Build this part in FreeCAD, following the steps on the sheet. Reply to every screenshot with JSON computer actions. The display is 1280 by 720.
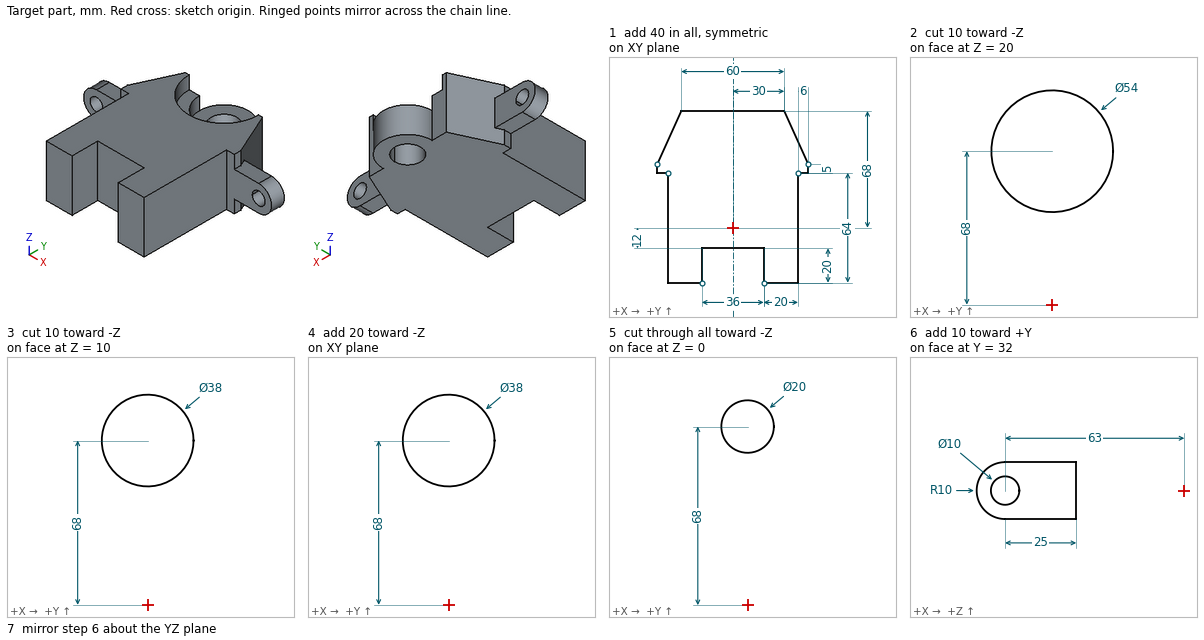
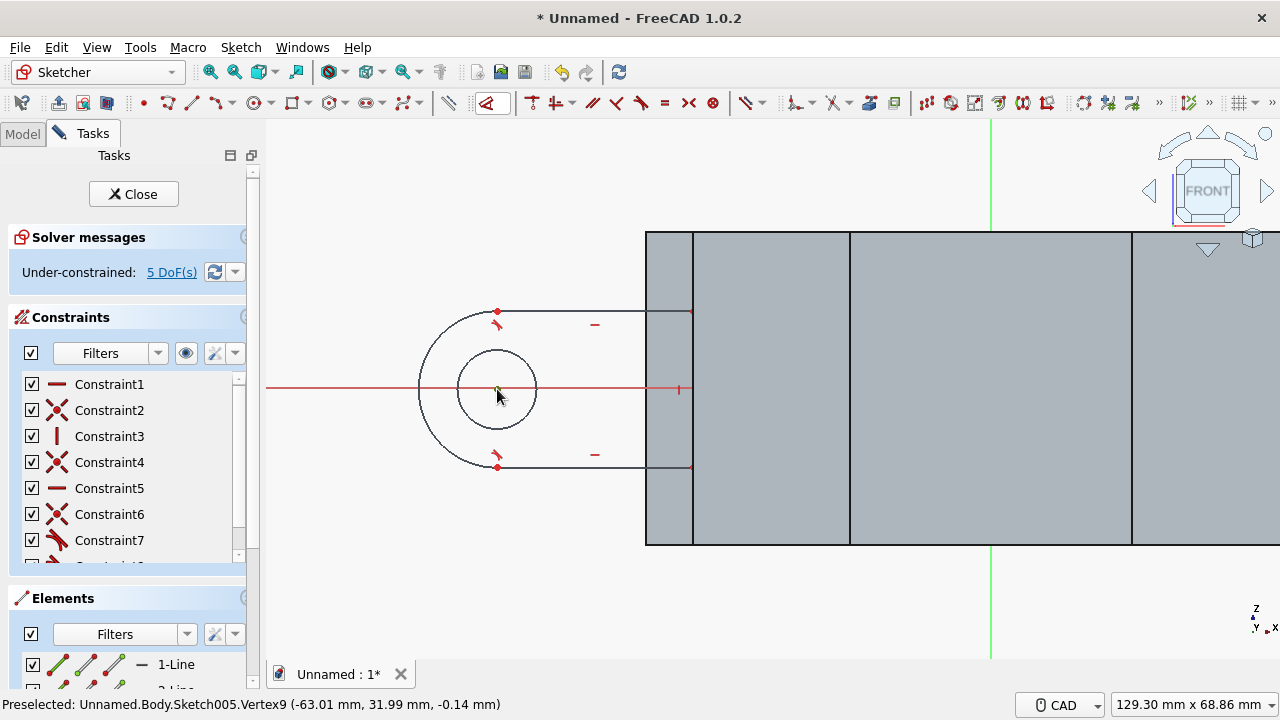
{"action": "left_click", "coordinate": [353, 388]}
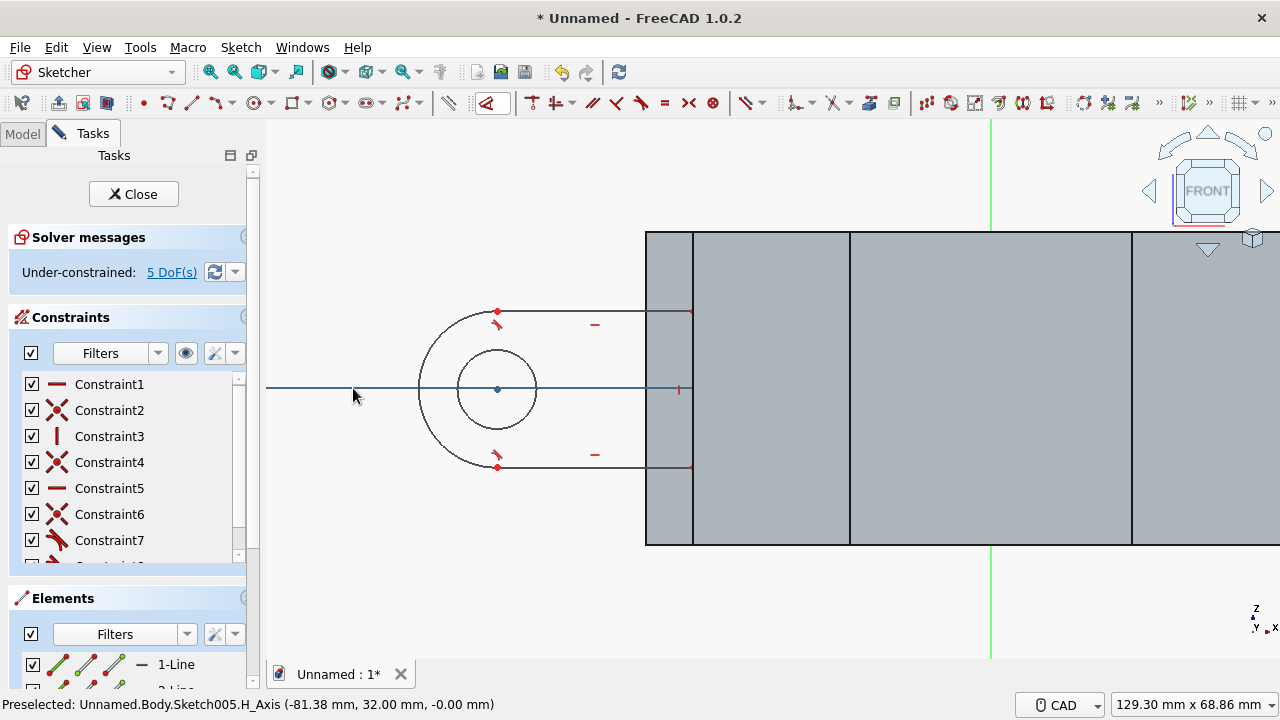
{"action": "left_click", "coordinate": [532, 104]}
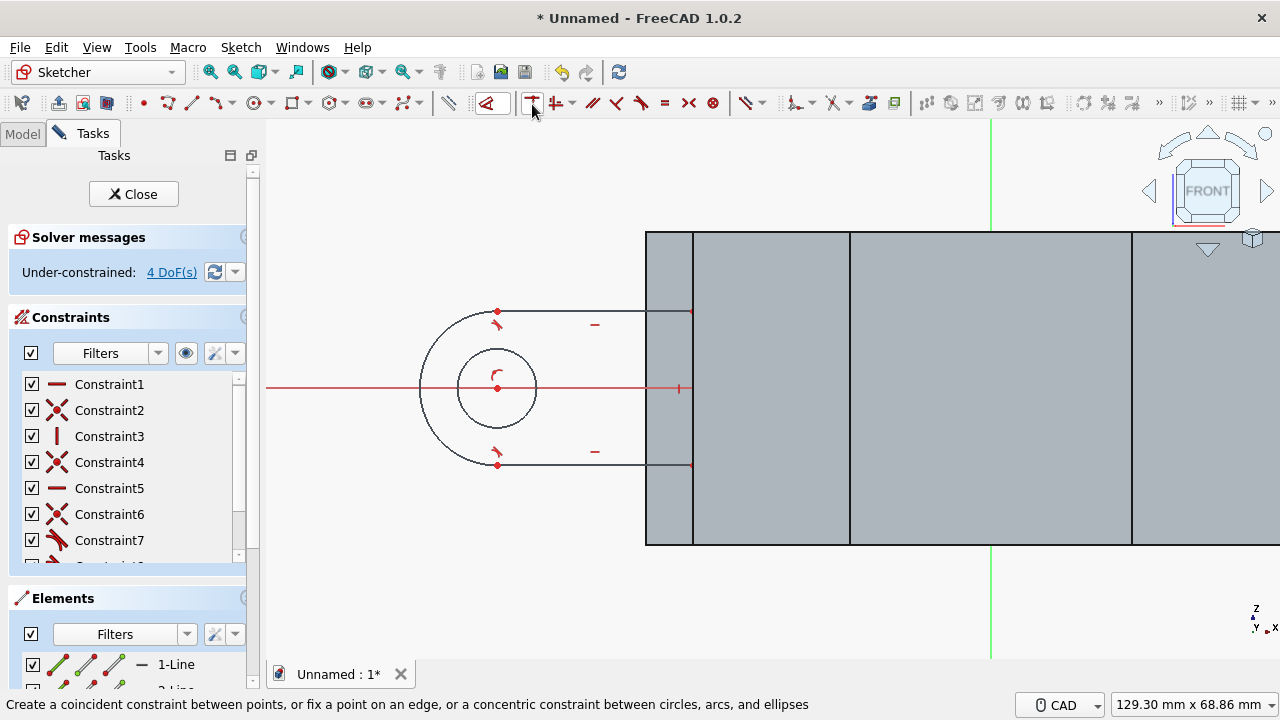
{"action": "left_click", "coordinate": [435, 343]}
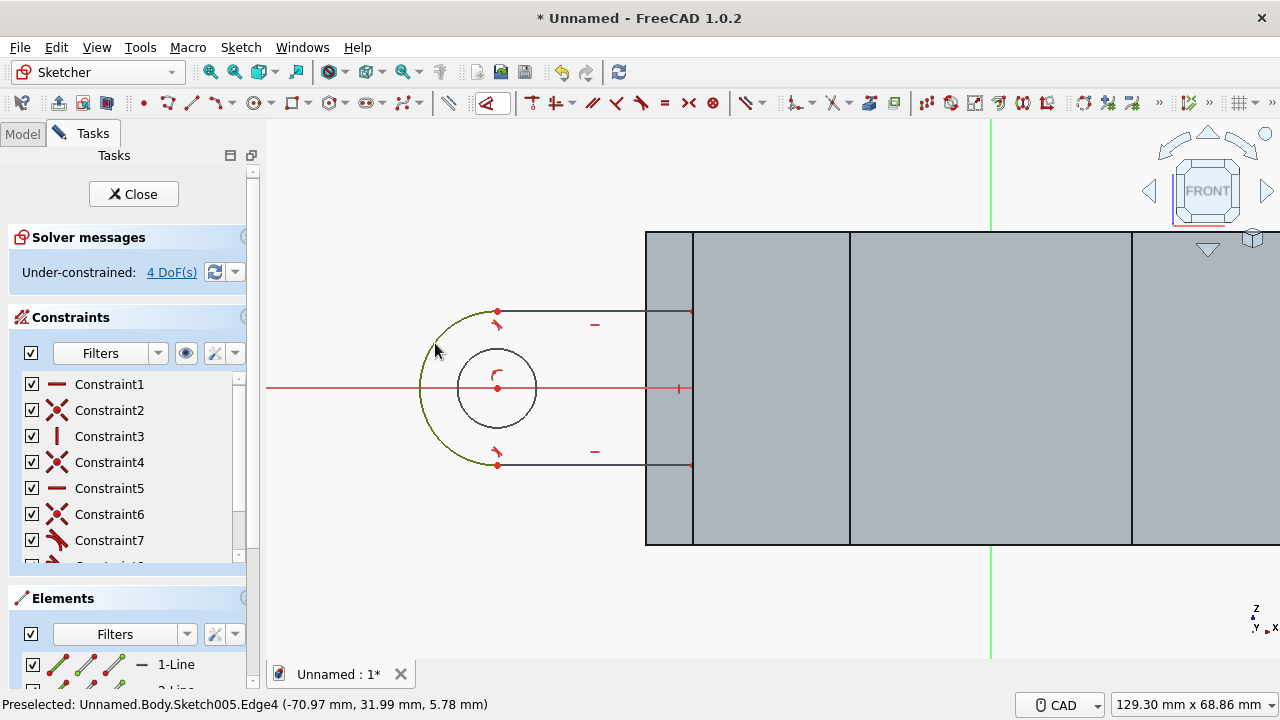
{"action": "left_click", "coordinate": [504, 104]}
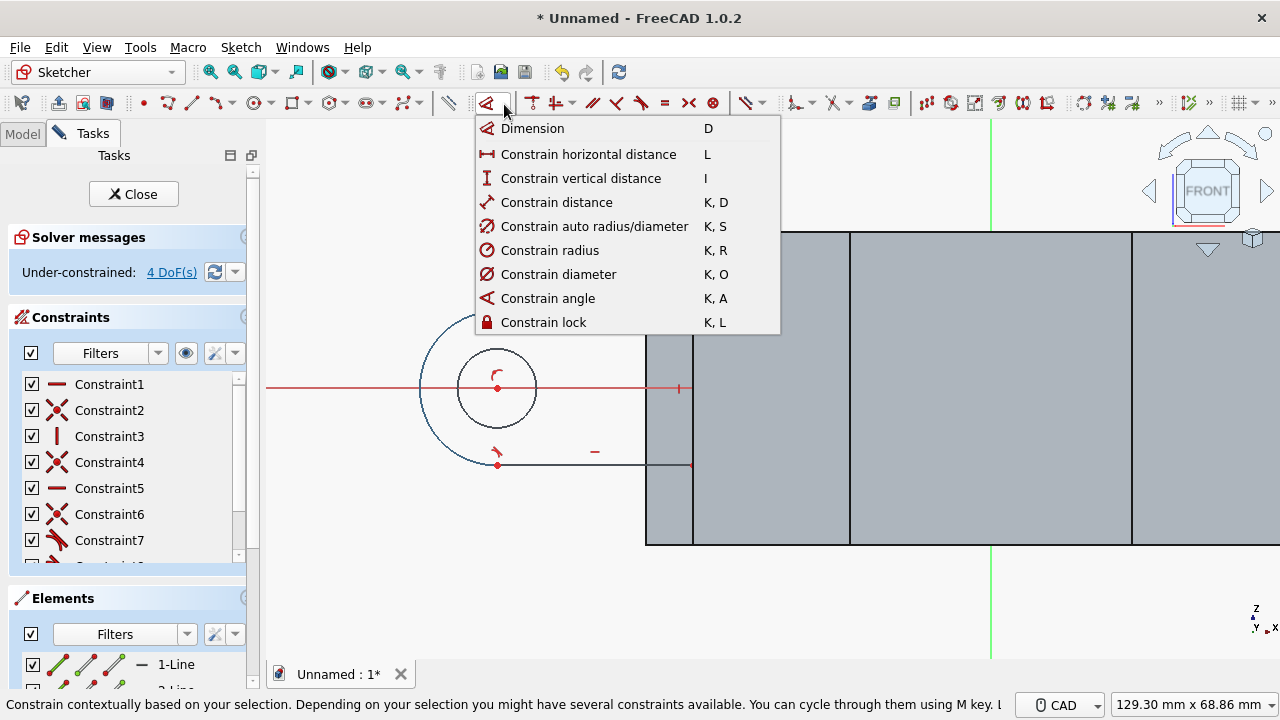
{"action": "left_click", "coordinate": [628, 250]}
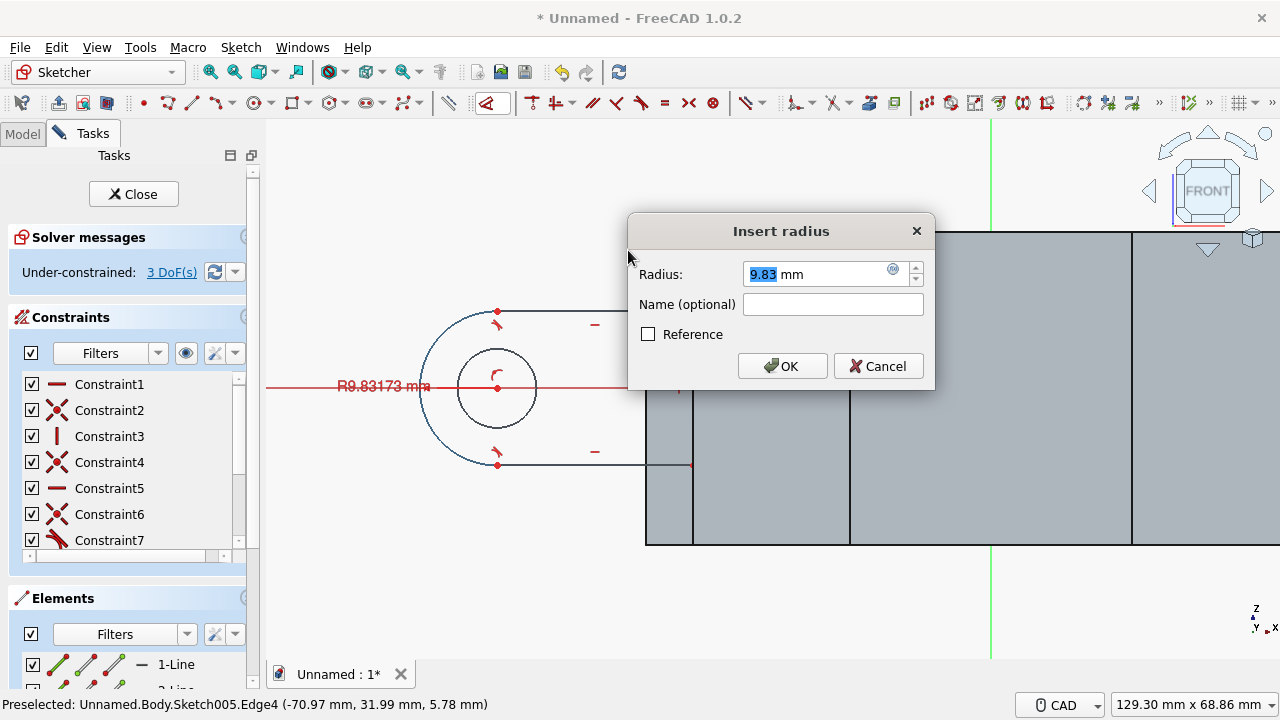
{"action": "type", "text": "10"}
{"action": "key", "text": "Return"}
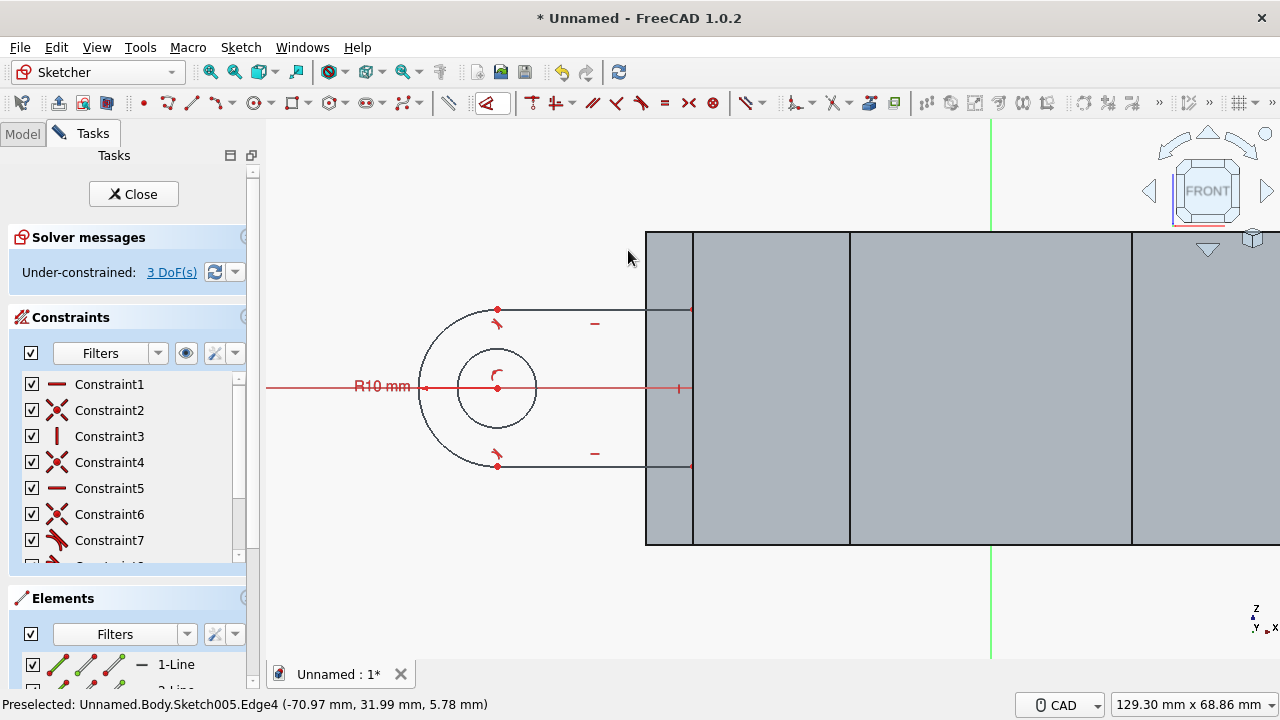
{"action": "left_click", "coordinate": [525, 360]}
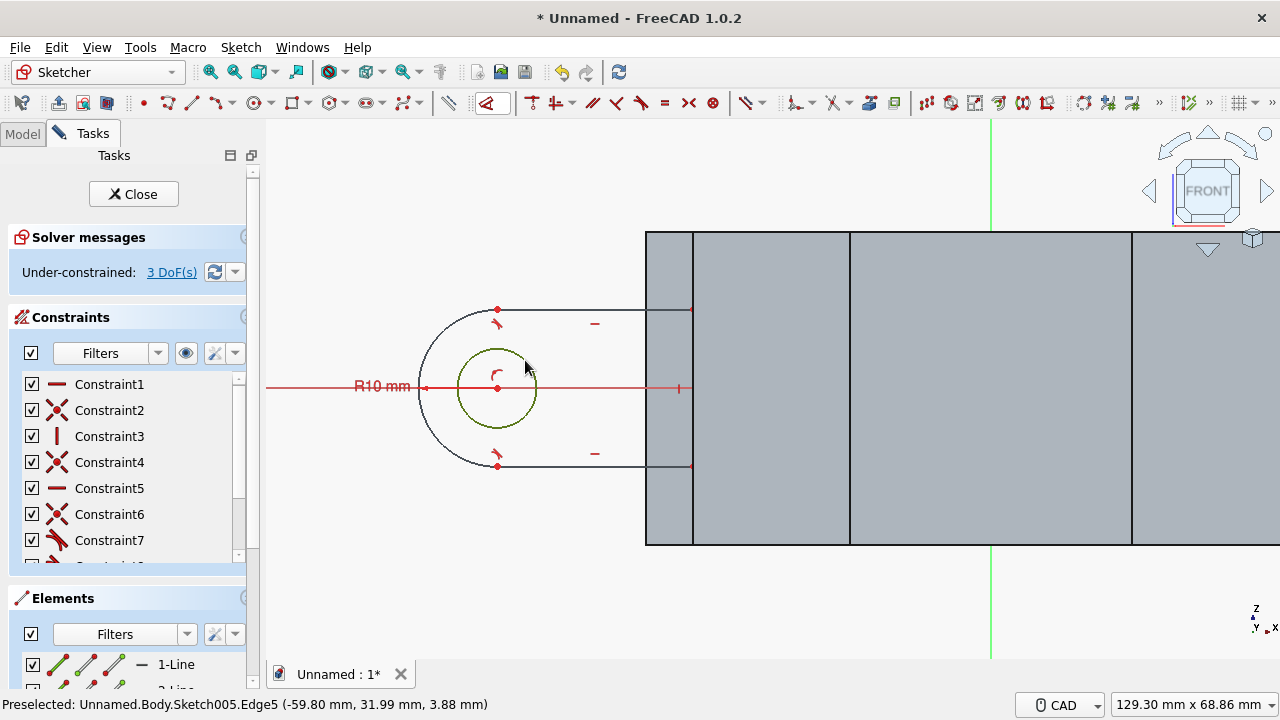
{"action": "key", "text": "k o"}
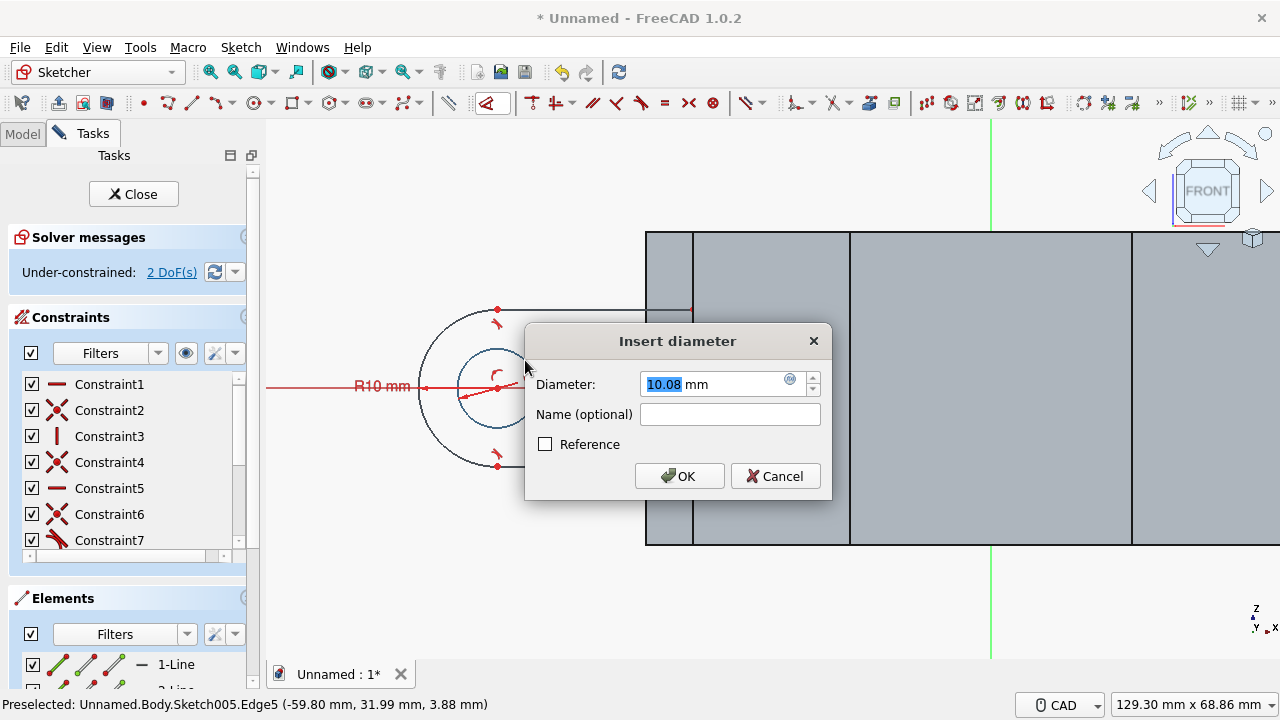
{"action": "type", "text": "10"}
{"action": "key", "text": "Return"}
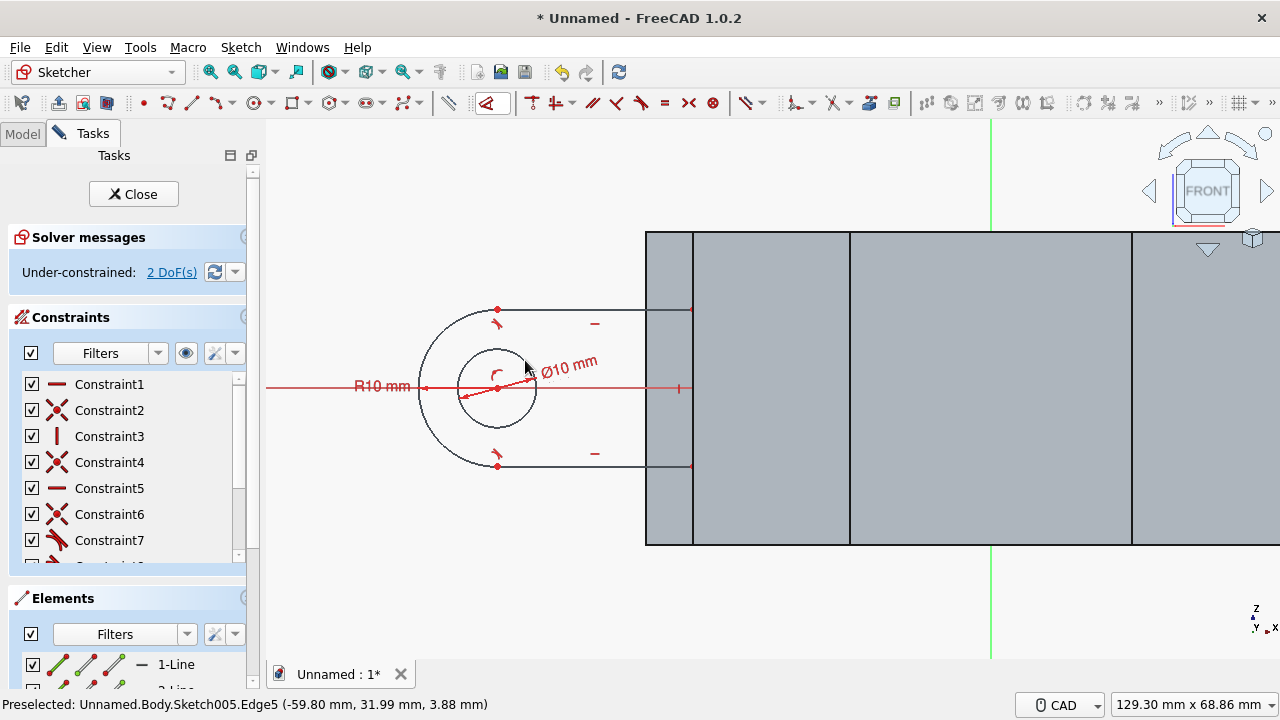
{"action": "left_click", "coordinate": [556, 467]}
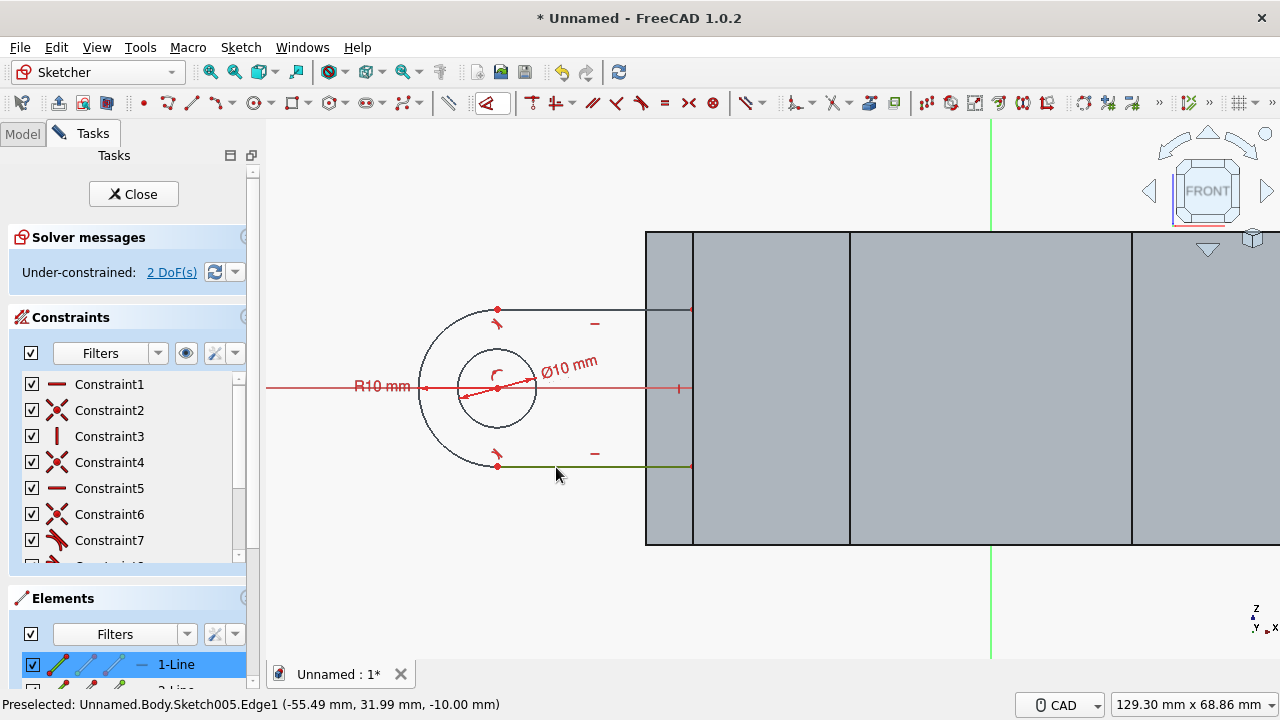
{"action": "key", "text": "l"}